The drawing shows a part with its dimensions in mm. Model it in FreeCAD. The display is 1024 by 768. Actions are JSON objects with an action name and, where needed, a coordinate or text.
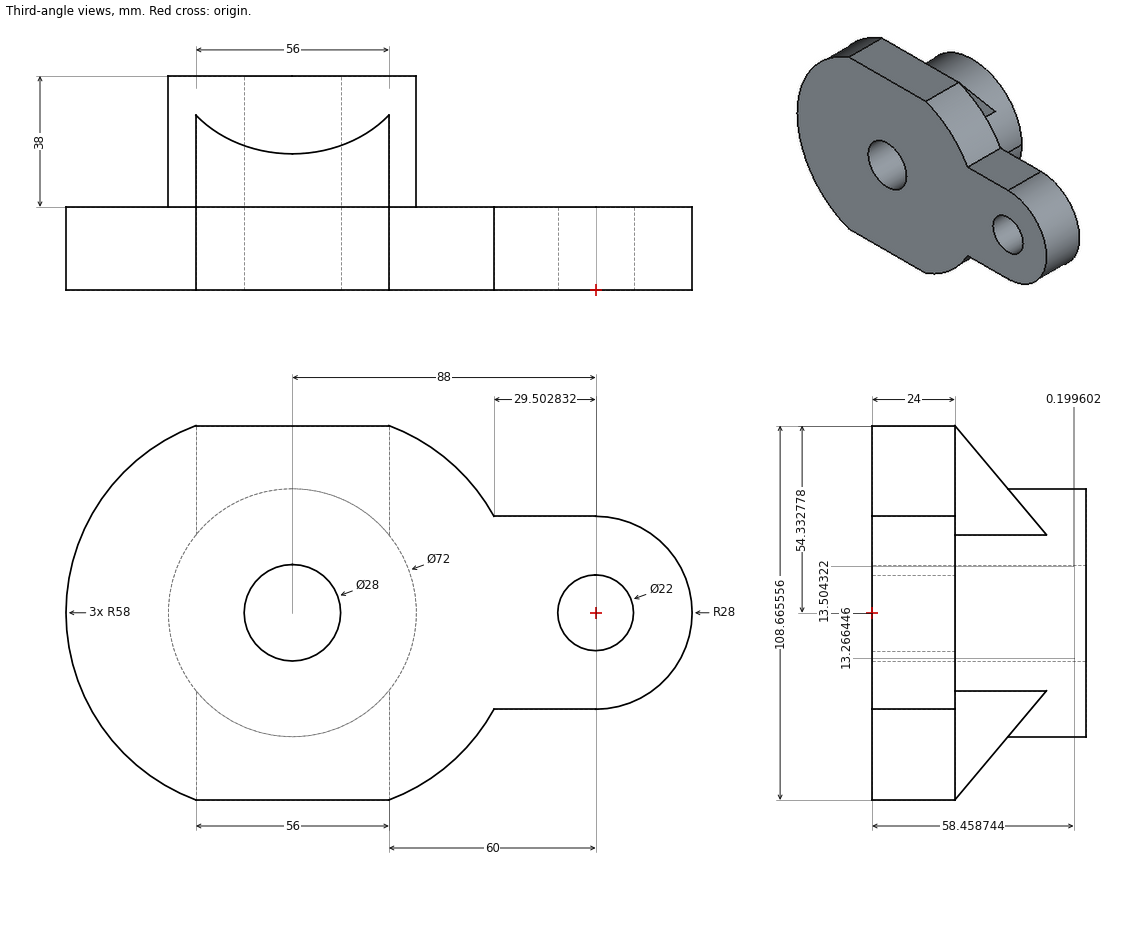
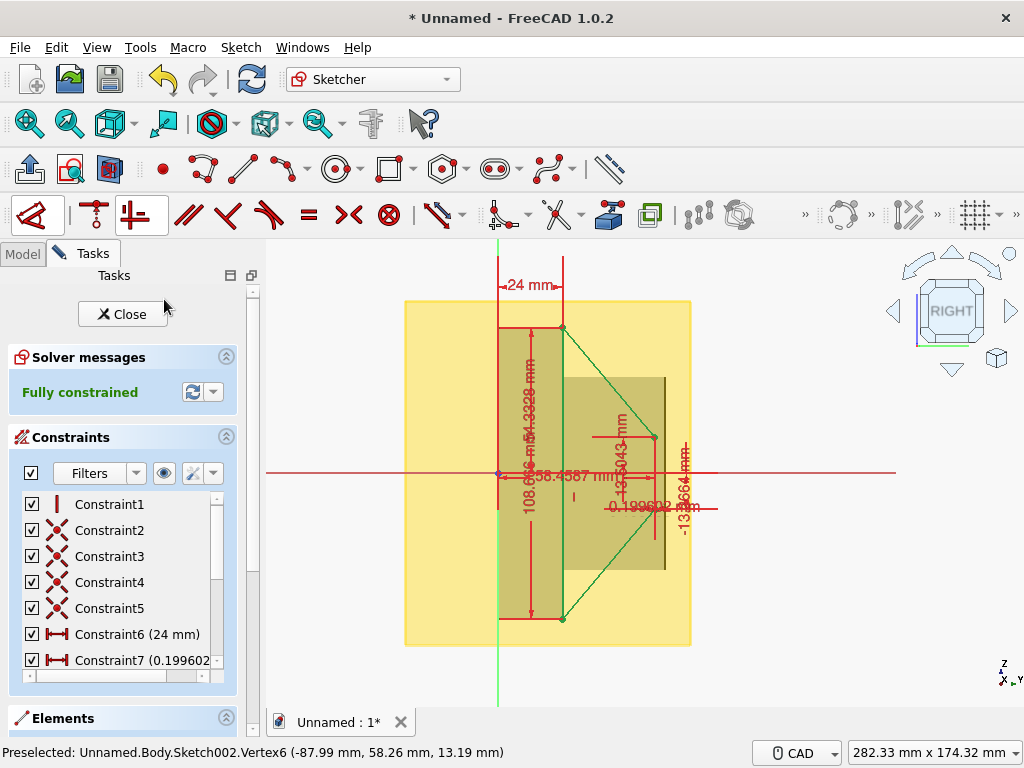
{"action": "left_click", "coordinate": [123, 314]}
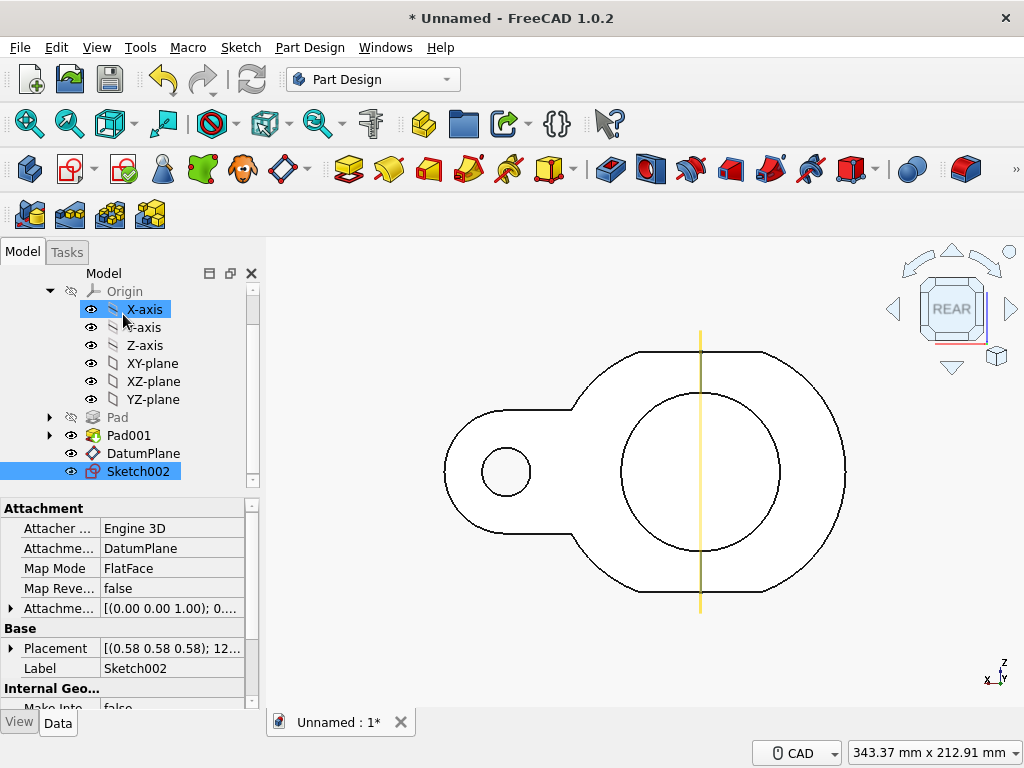
{"action": "left_click", "coordinate": [350, 170]}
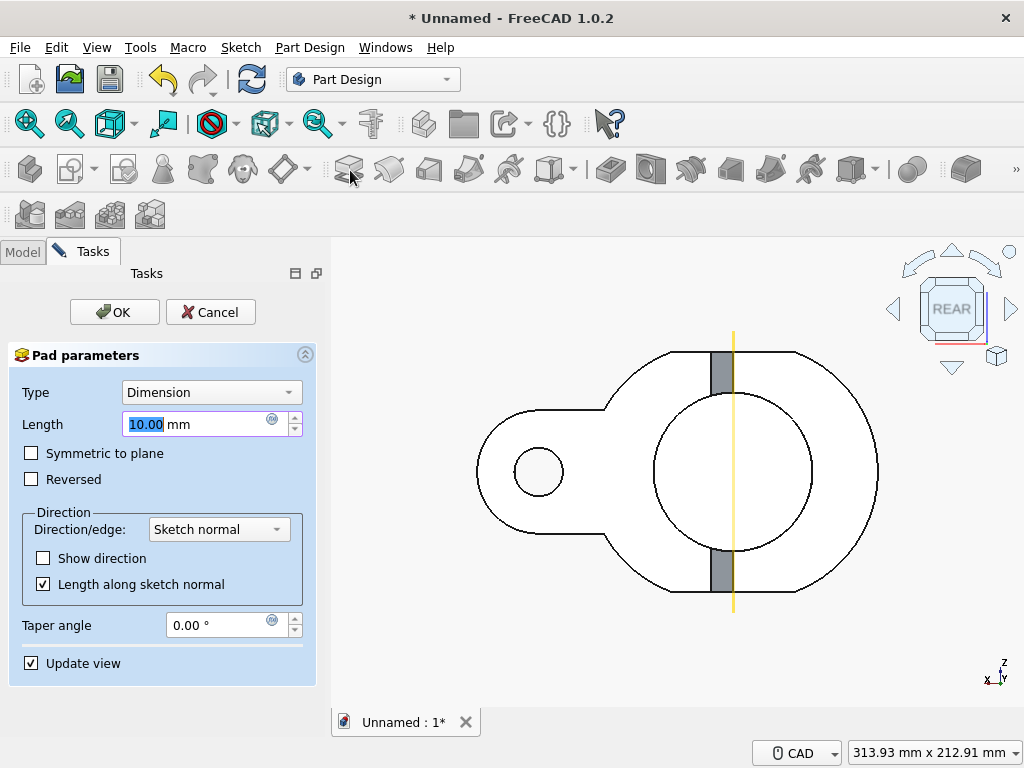
{"action": "type", "text": "56"}
{"action": "key", "text": "Tab"}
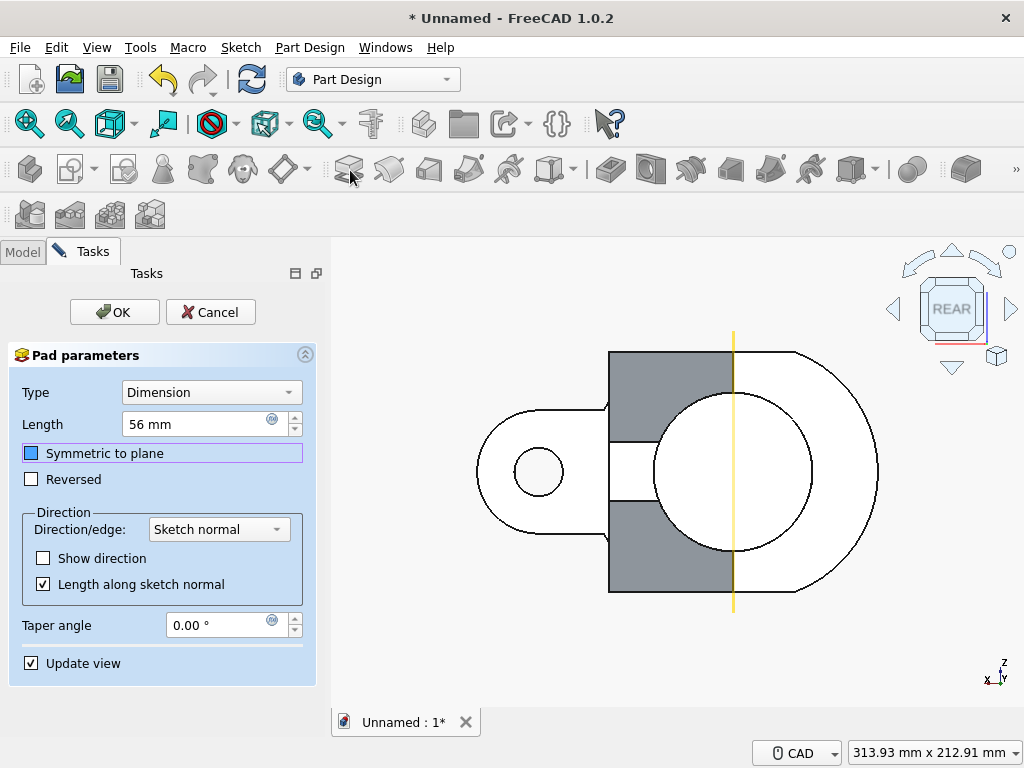
{"action": "left_click", "coordinate": [30, 453]}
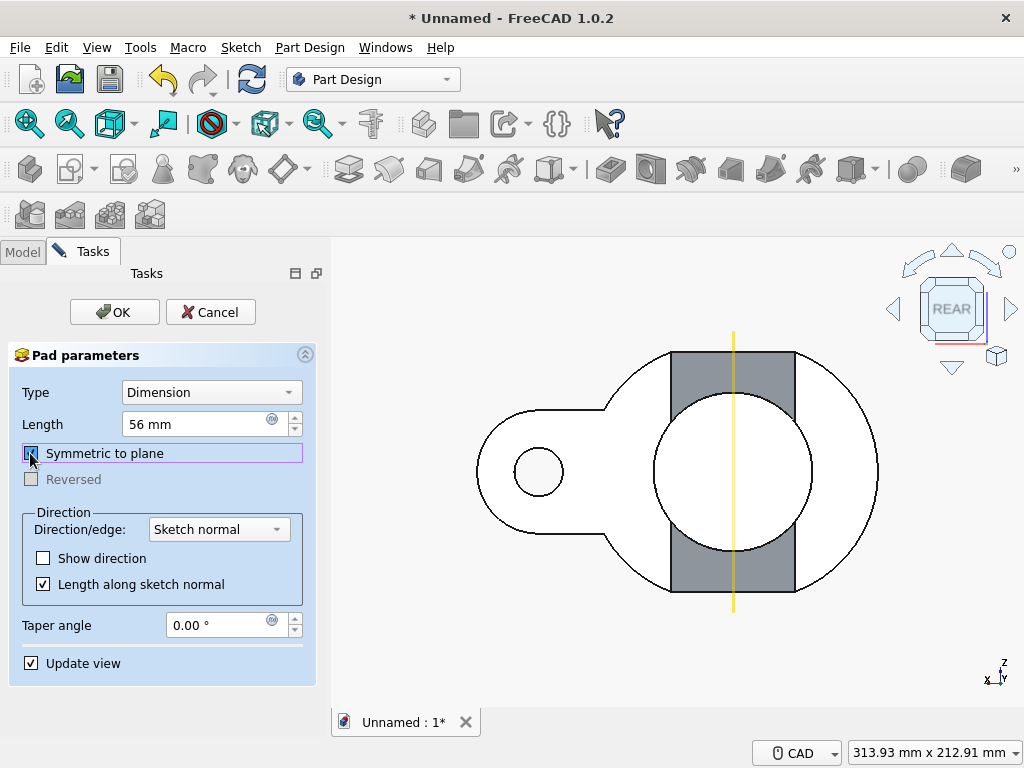
{"action": "left_click", "coordinate": [115, 312]}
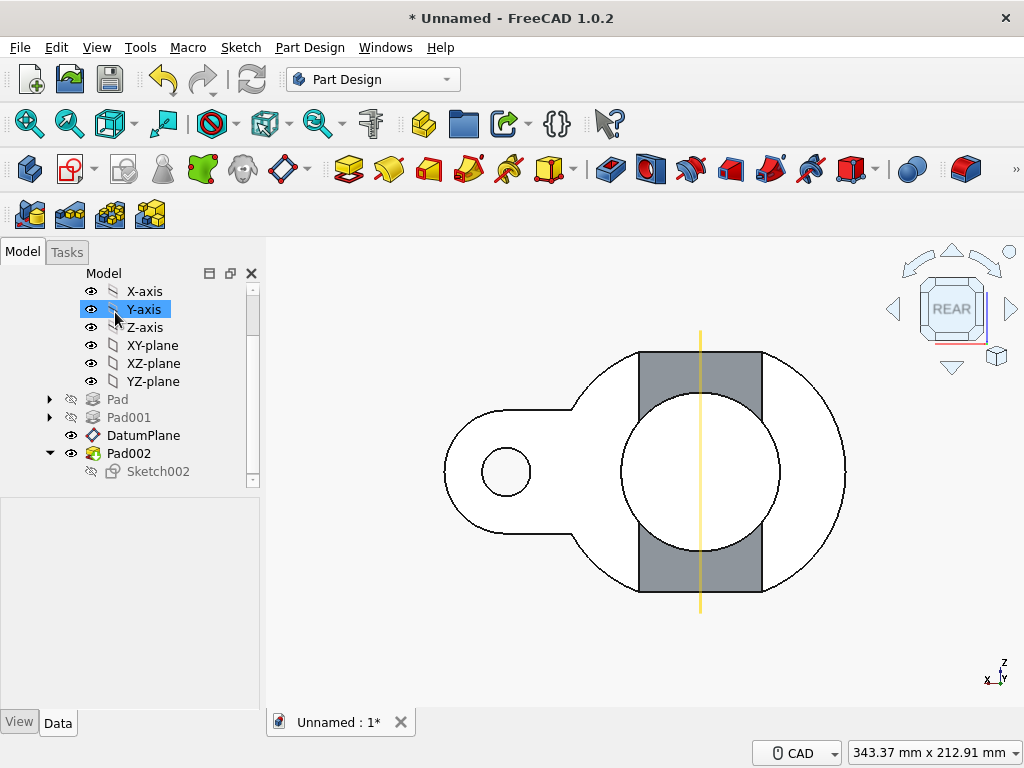
{"action": "left_click", "coordinate": [116, 435]}
{"action": "key", "text": "space"}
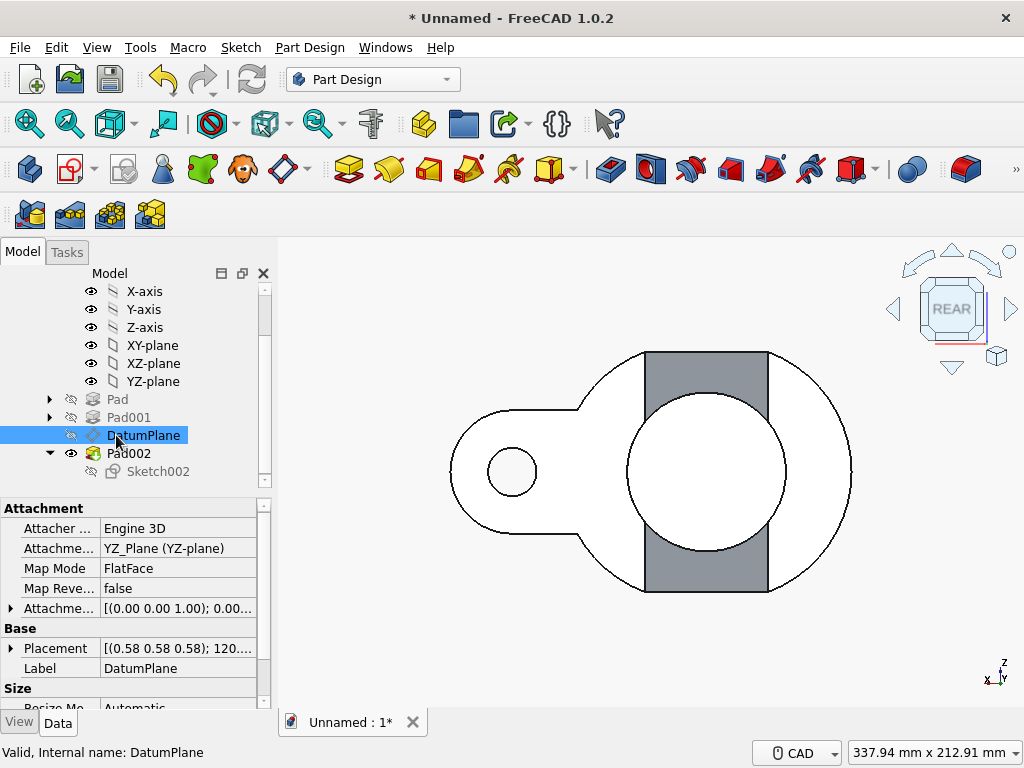
{"action": "left_click", "coordinate": [707, 471]}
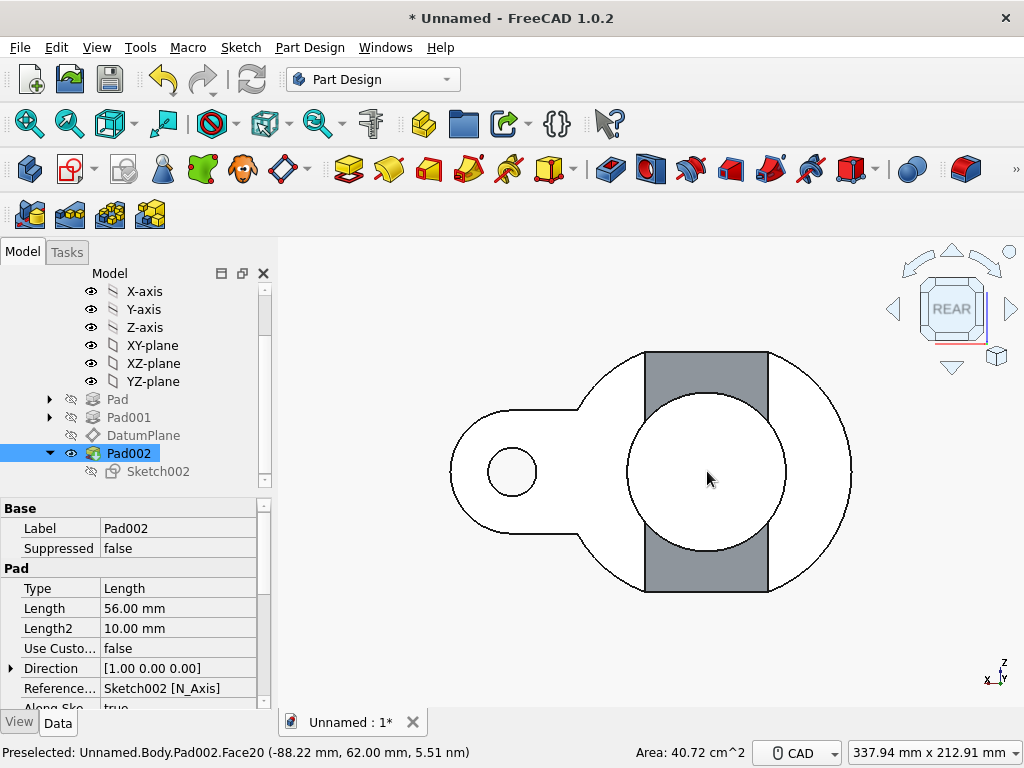
{"action": "left_click", "coordinate": [70, 170]}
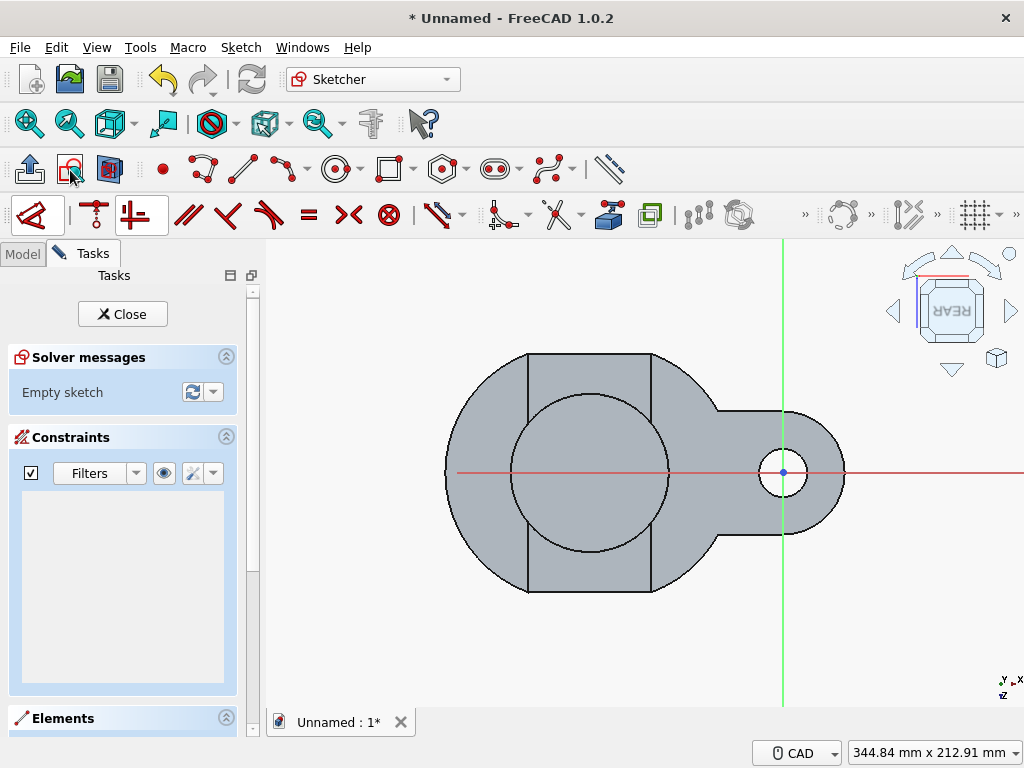
{"action": "scroll", "coordinate": [593, 473], "scroll_direction": "up", "scroll_amount": 8}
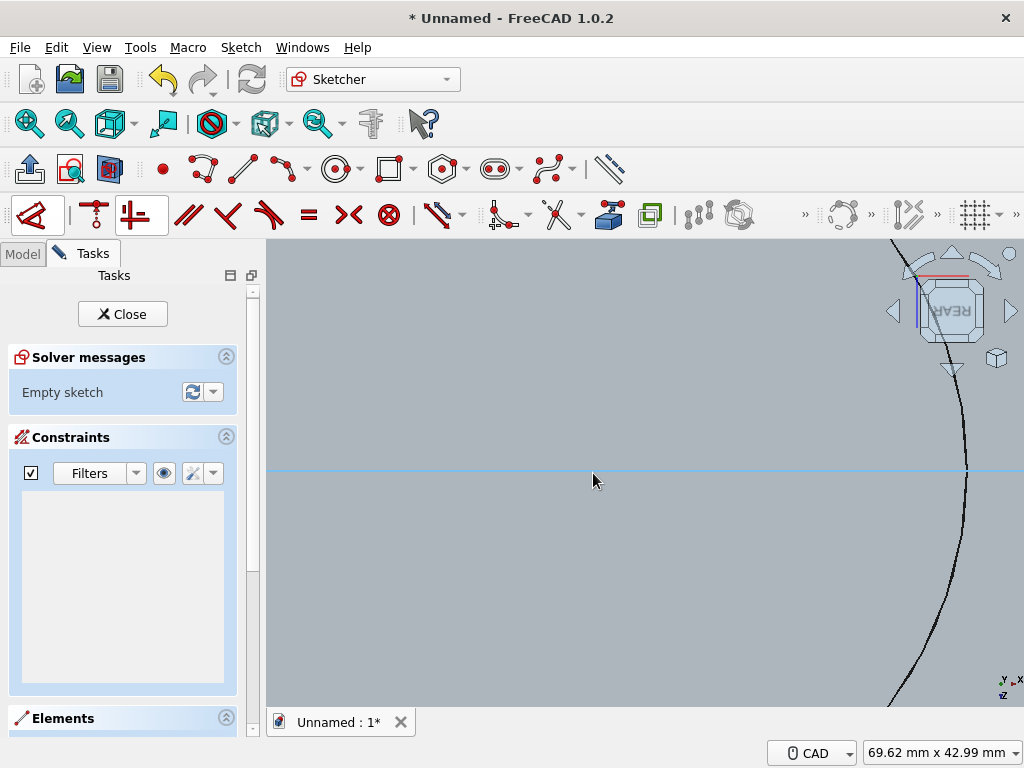
{"action": "left_click", "coordinate": [336, 170]}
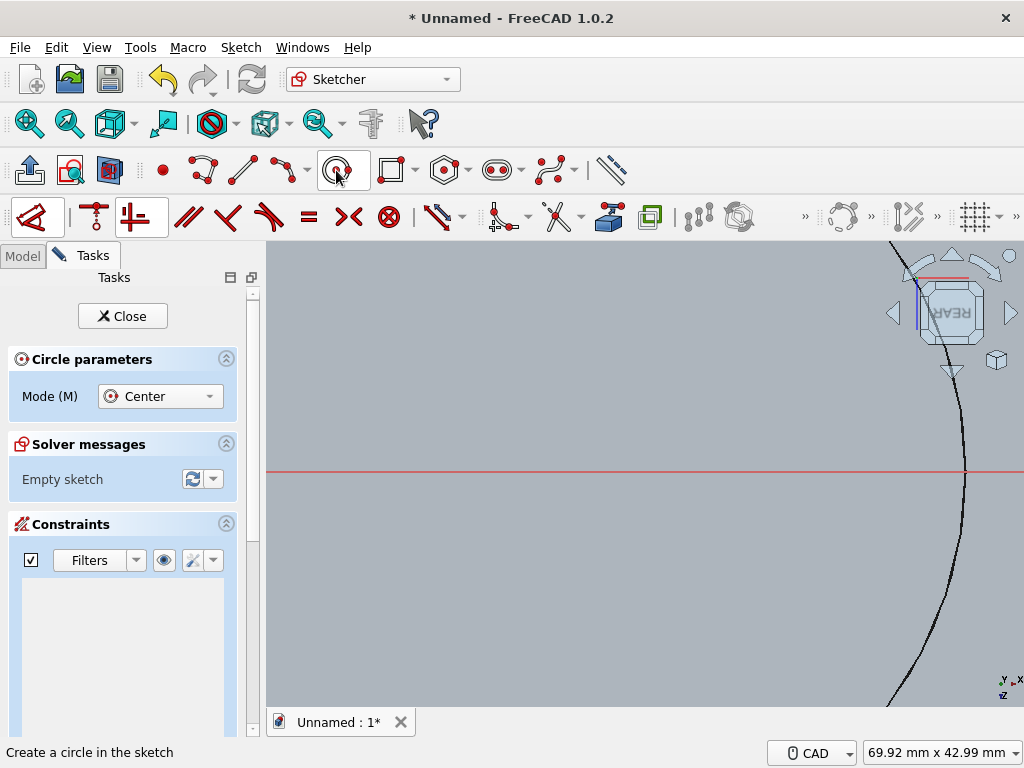
{"action": "left_click", "coordinate": [575, 472]}
{"action": "mouse_move", "coordinate": [683, 365]}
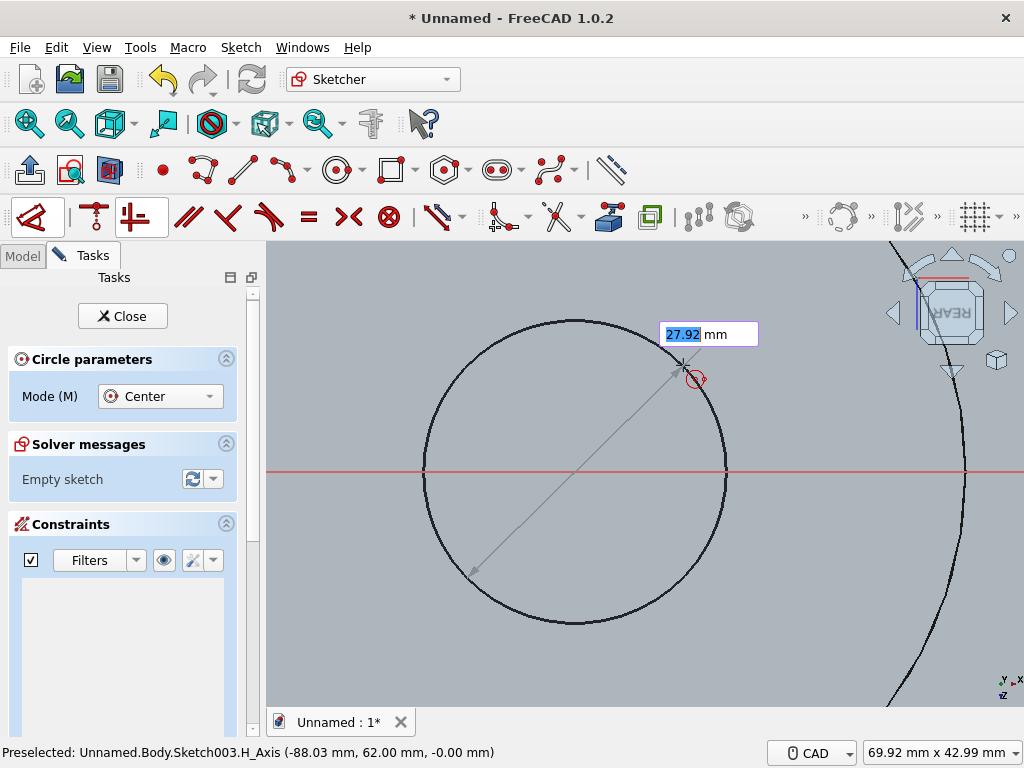
{"action": "type", "text": "28"}
{"action": "key", "text": "Return"}
{"action": "key", "text": "Escape"}